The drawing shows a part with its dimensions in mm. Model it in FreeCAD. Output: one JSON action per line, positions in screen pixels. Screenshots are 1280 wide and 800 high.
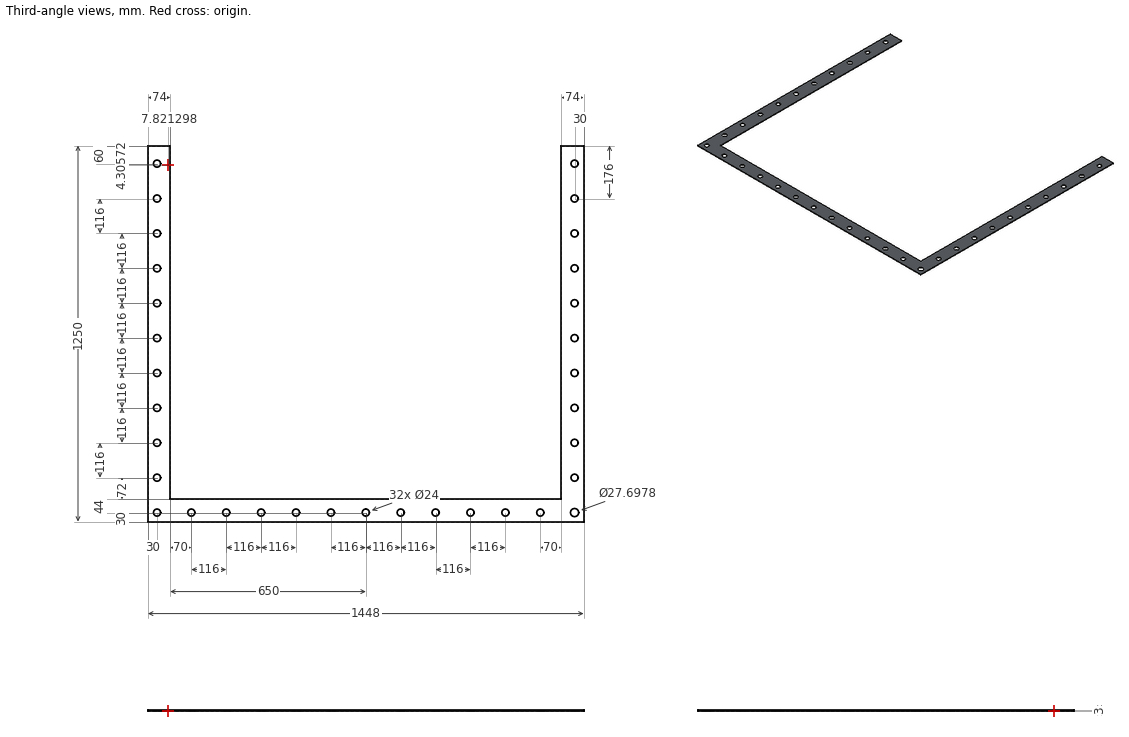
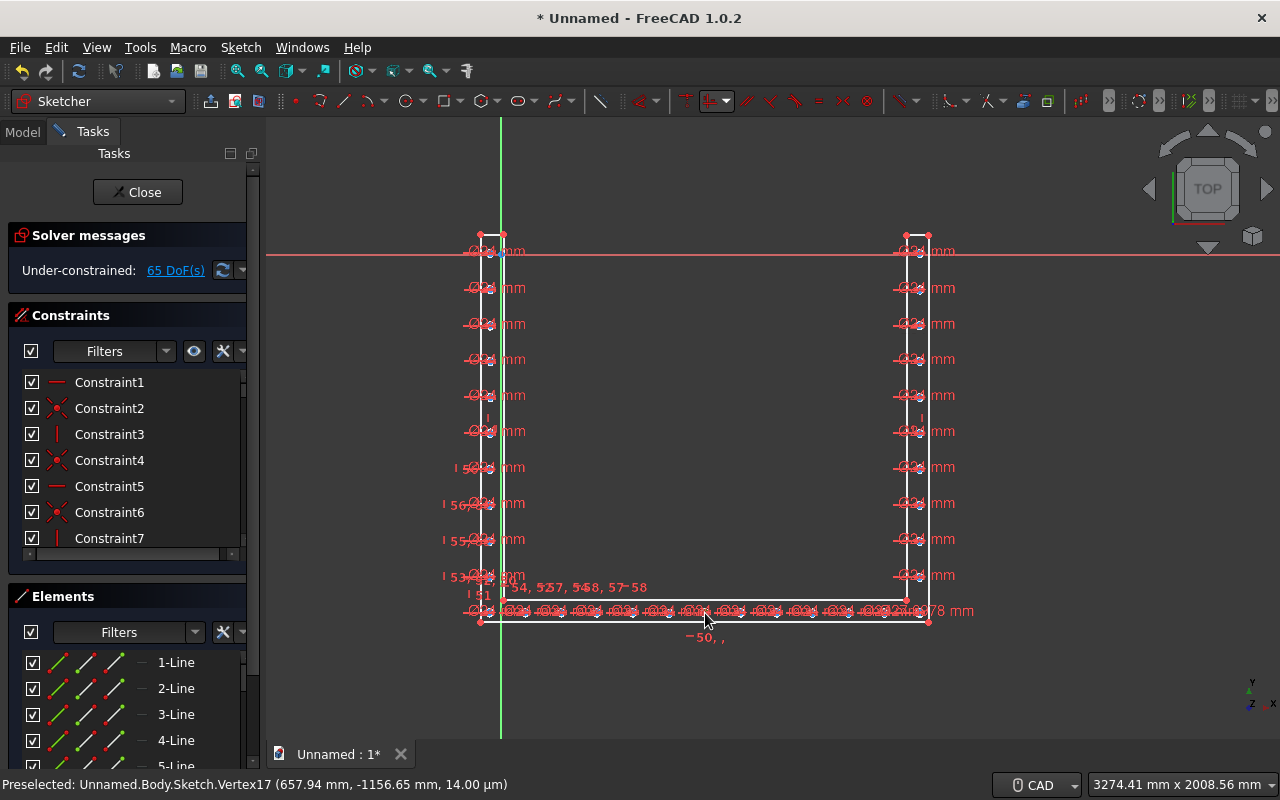
{"action": "left_click", "coordinate": [669, 613]}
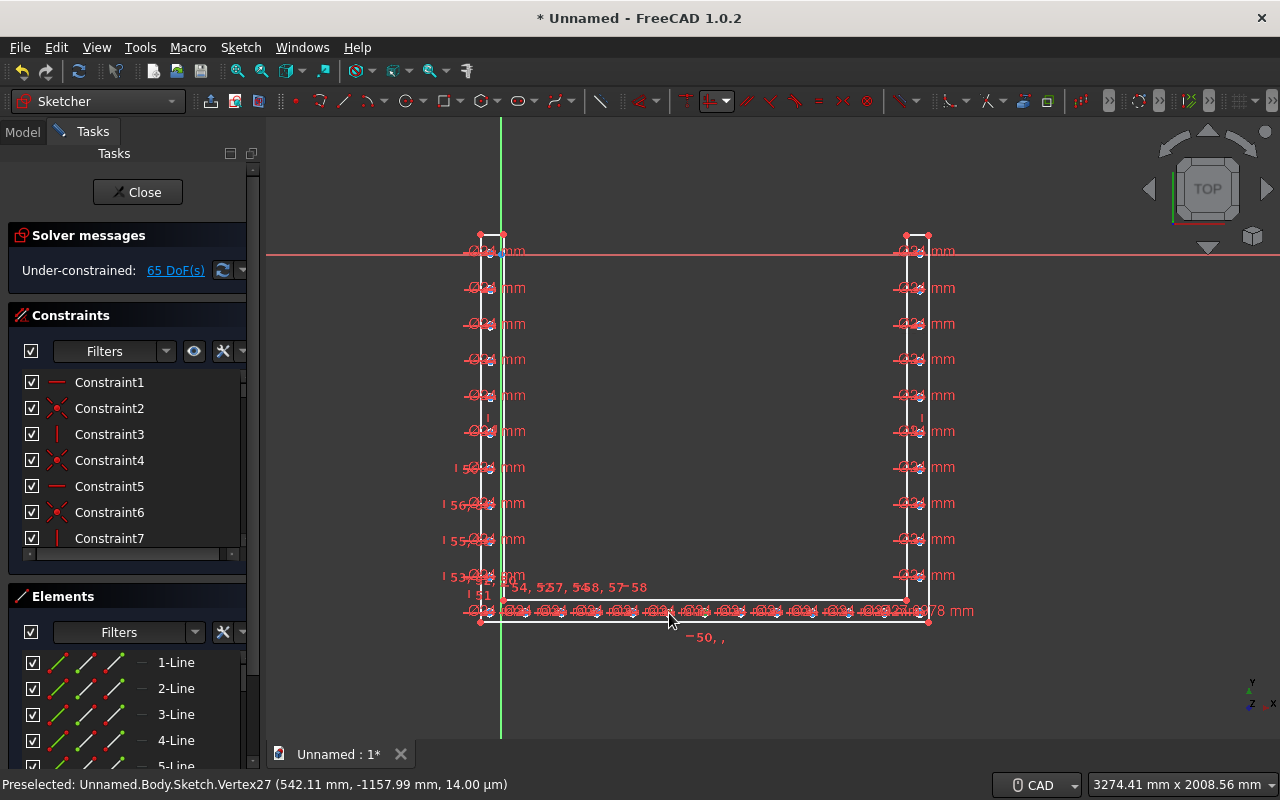
{"action": "left_click", "coordinate": [728, 102]}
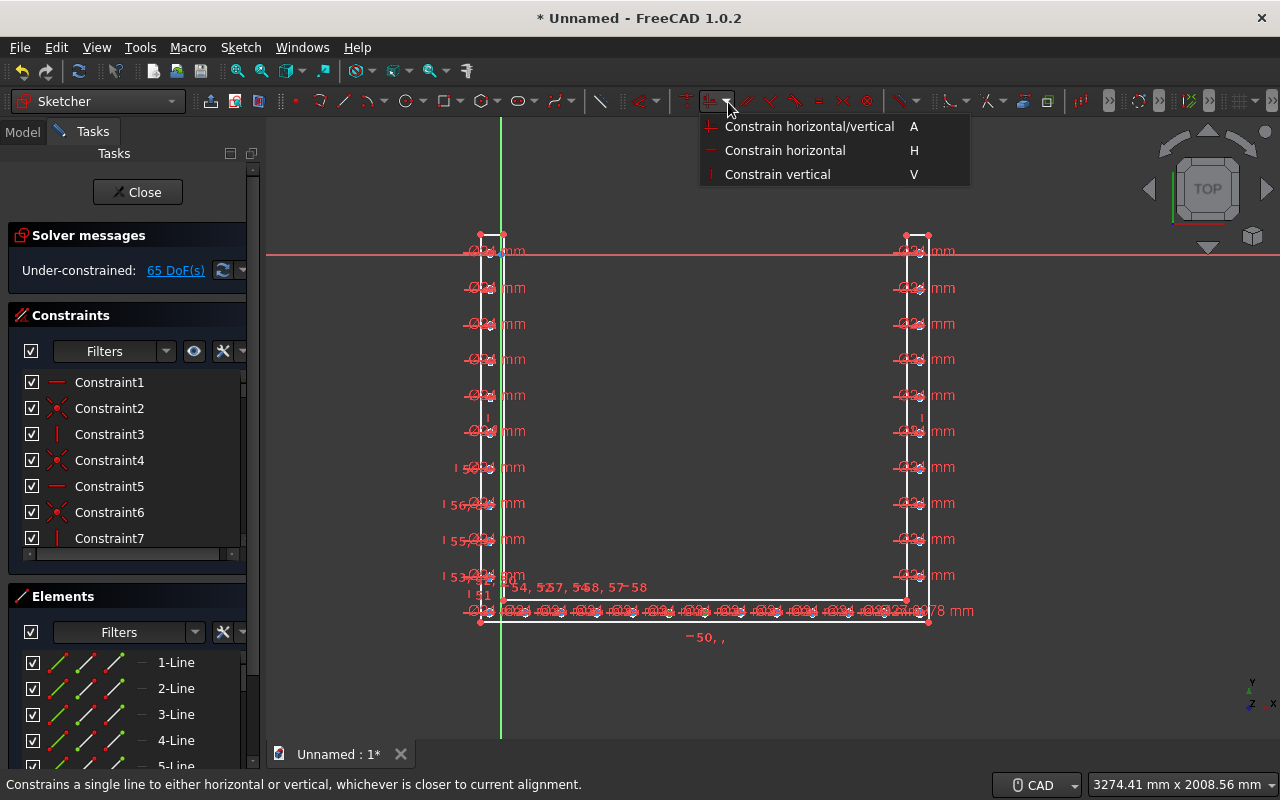
{"action": "left_click", "coordinate": [835, 150]}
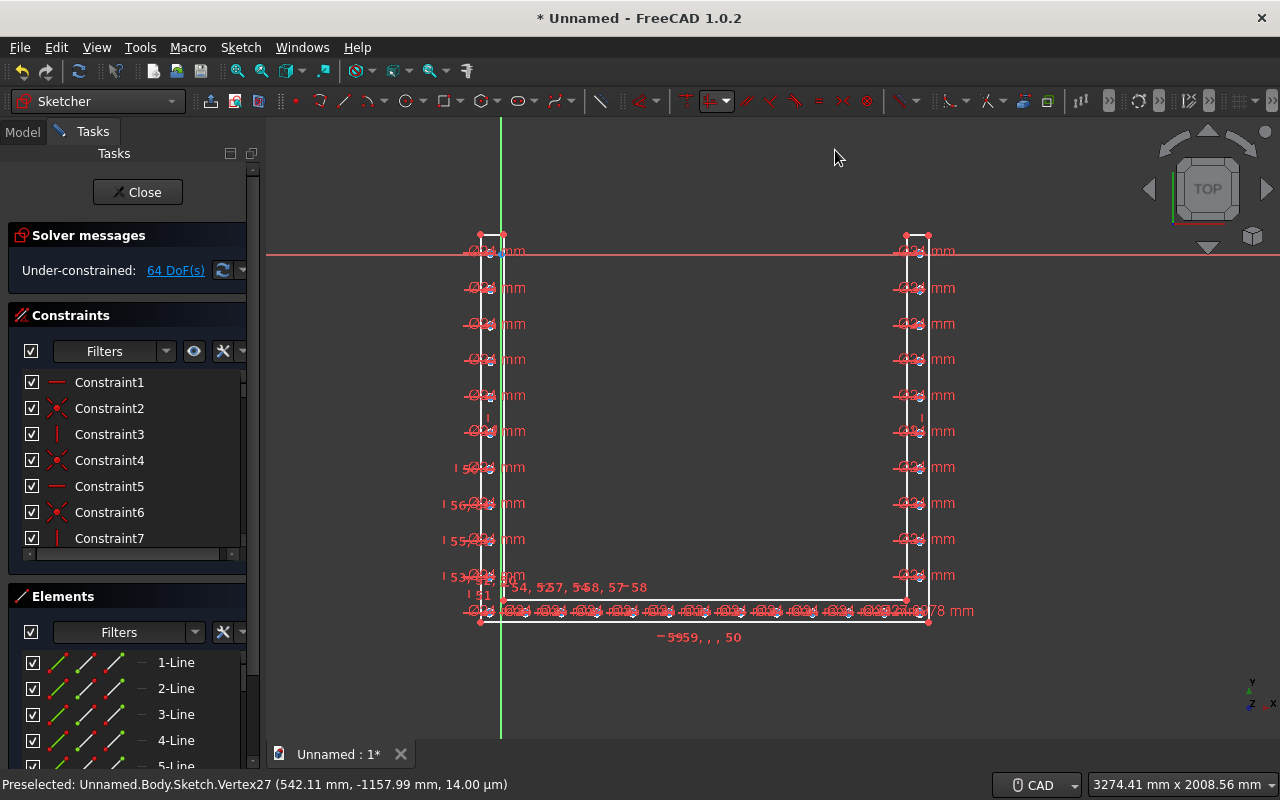
{"action": "left_click", "coordinate": [490, 469]}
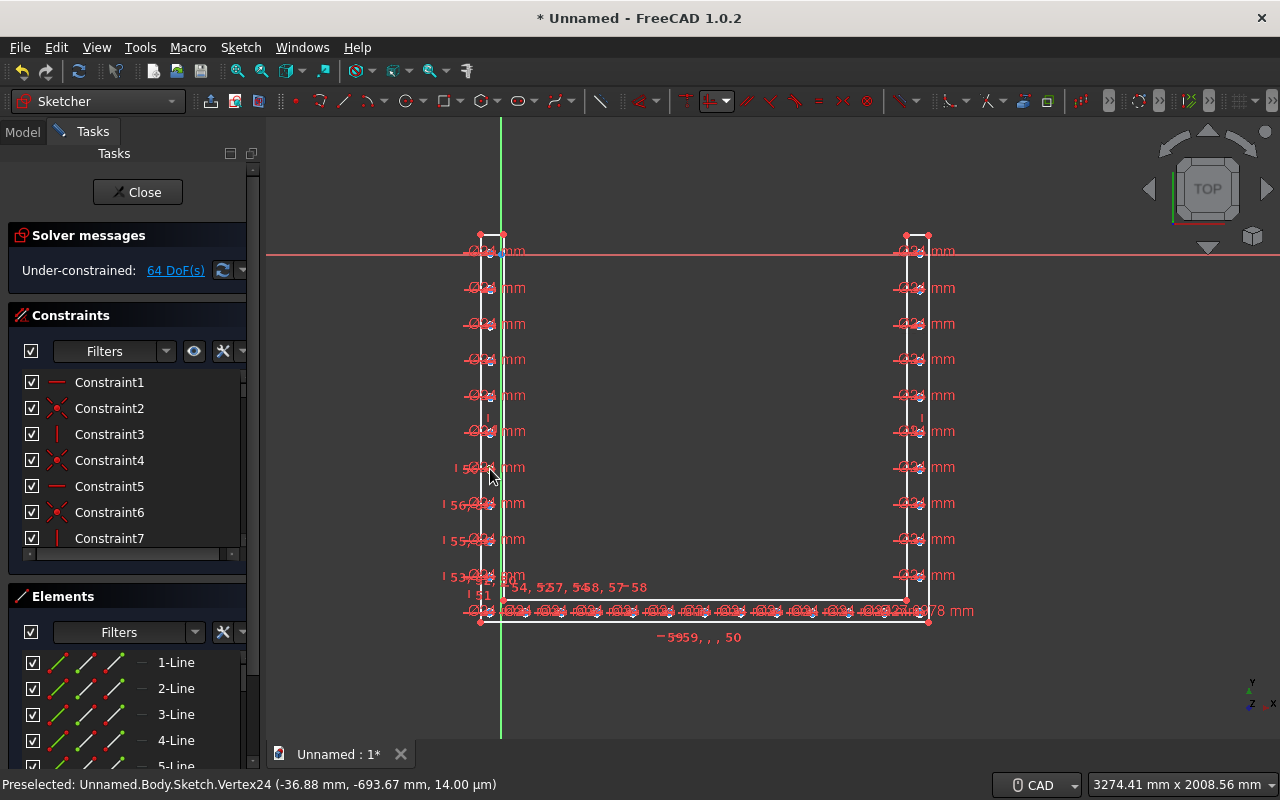
{"action": "left_click", "coordinate": [490, 433]}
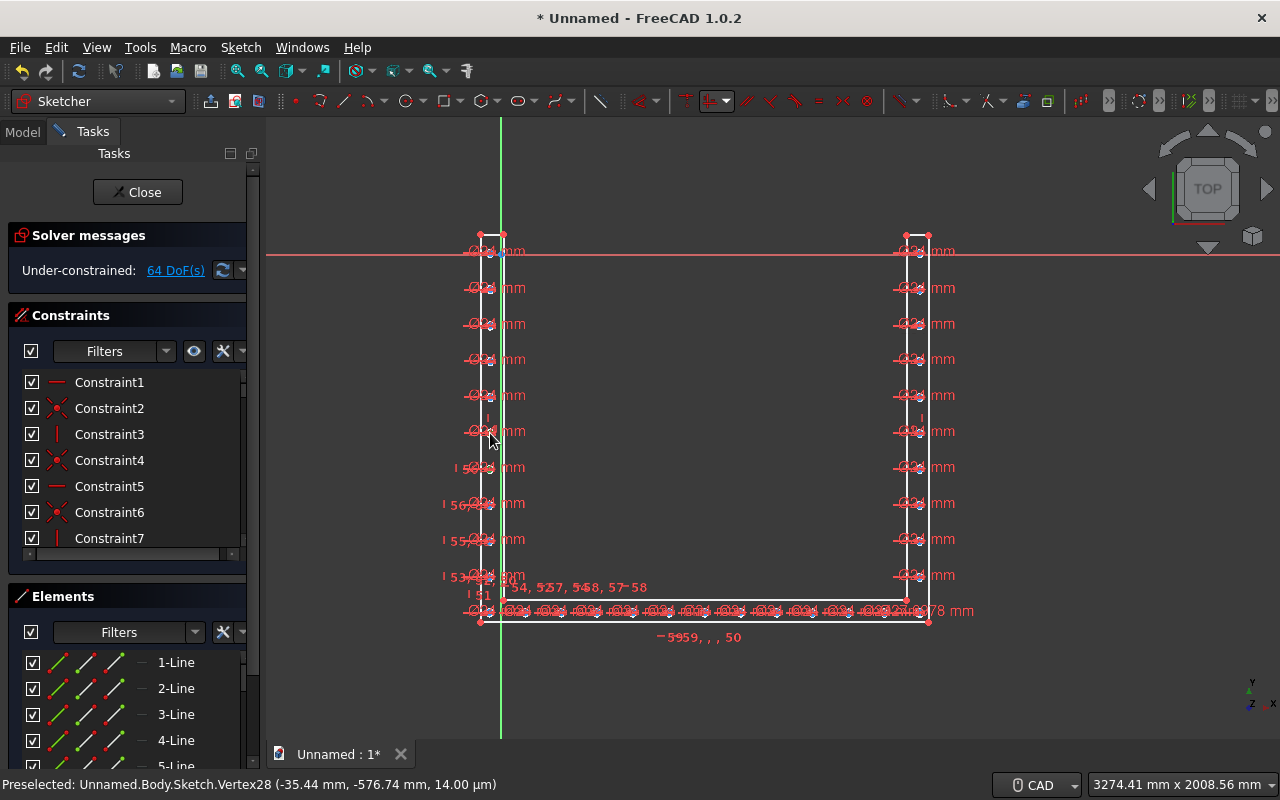
{"action": "key", "text": "v"}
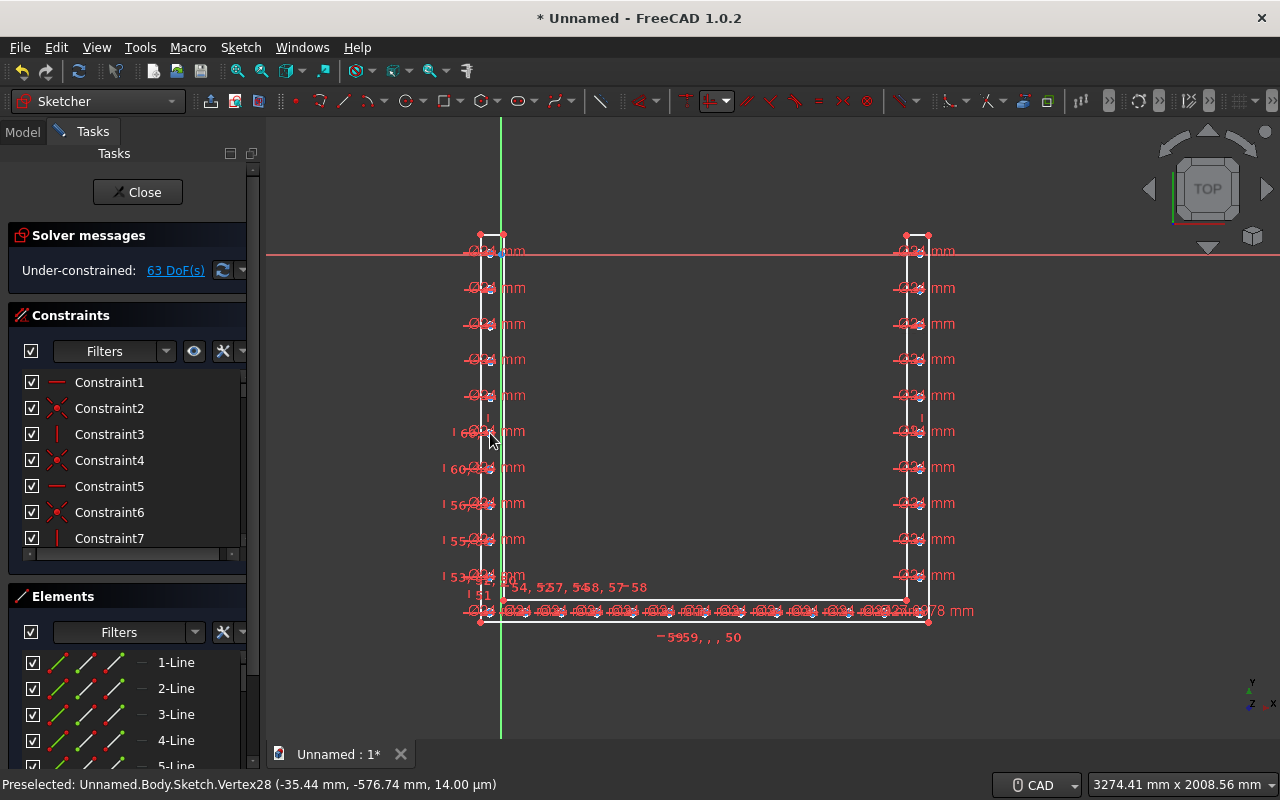
{"action": "left_click", "coordinate": [490, 433]}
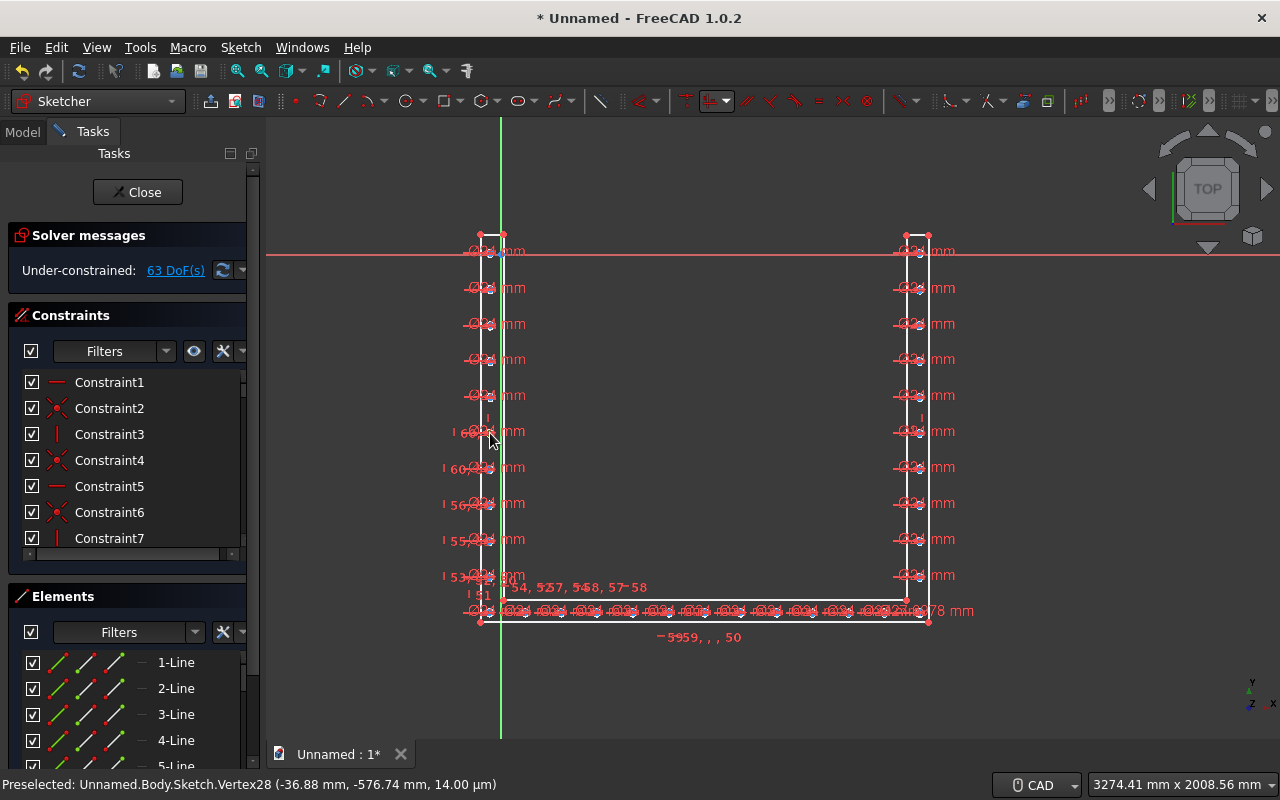
{"action": "left_click", "coordinate": [490, 397]}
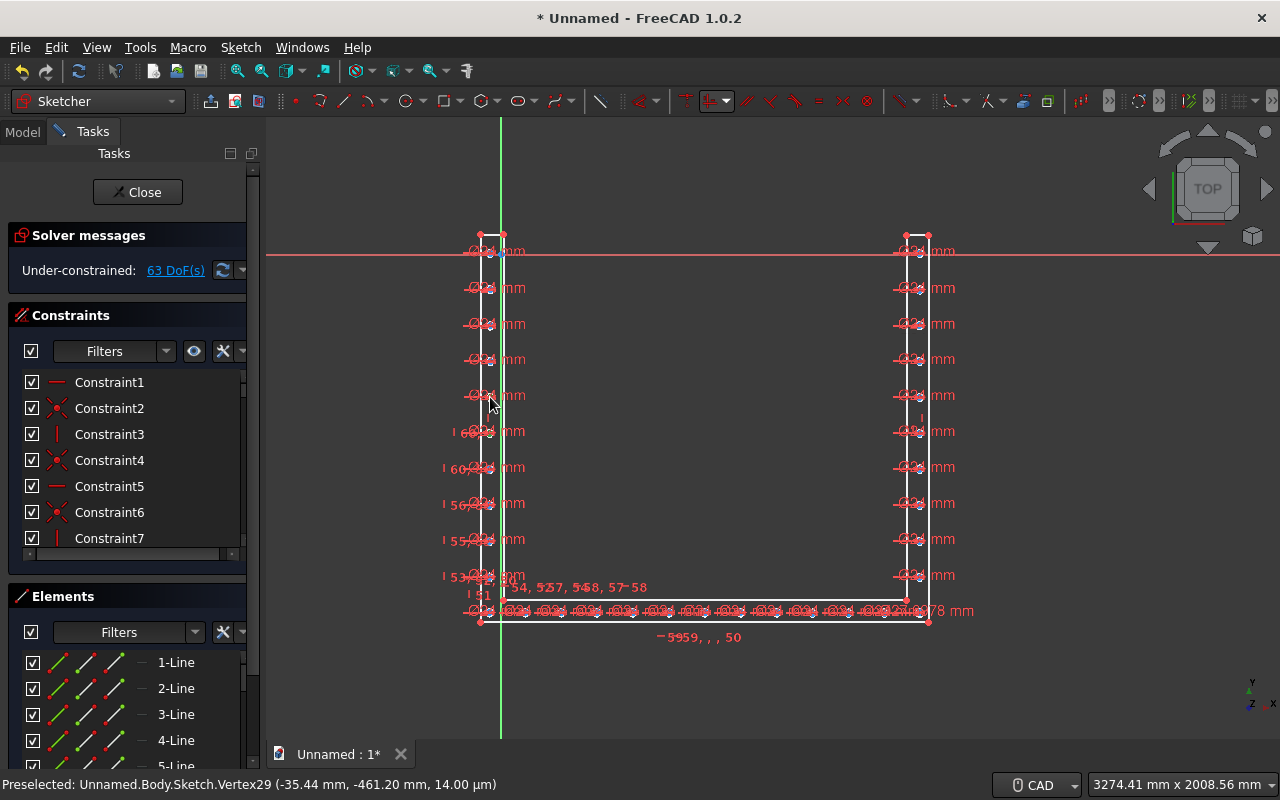
{"action": "left_click", "coordinate": [728, 102]}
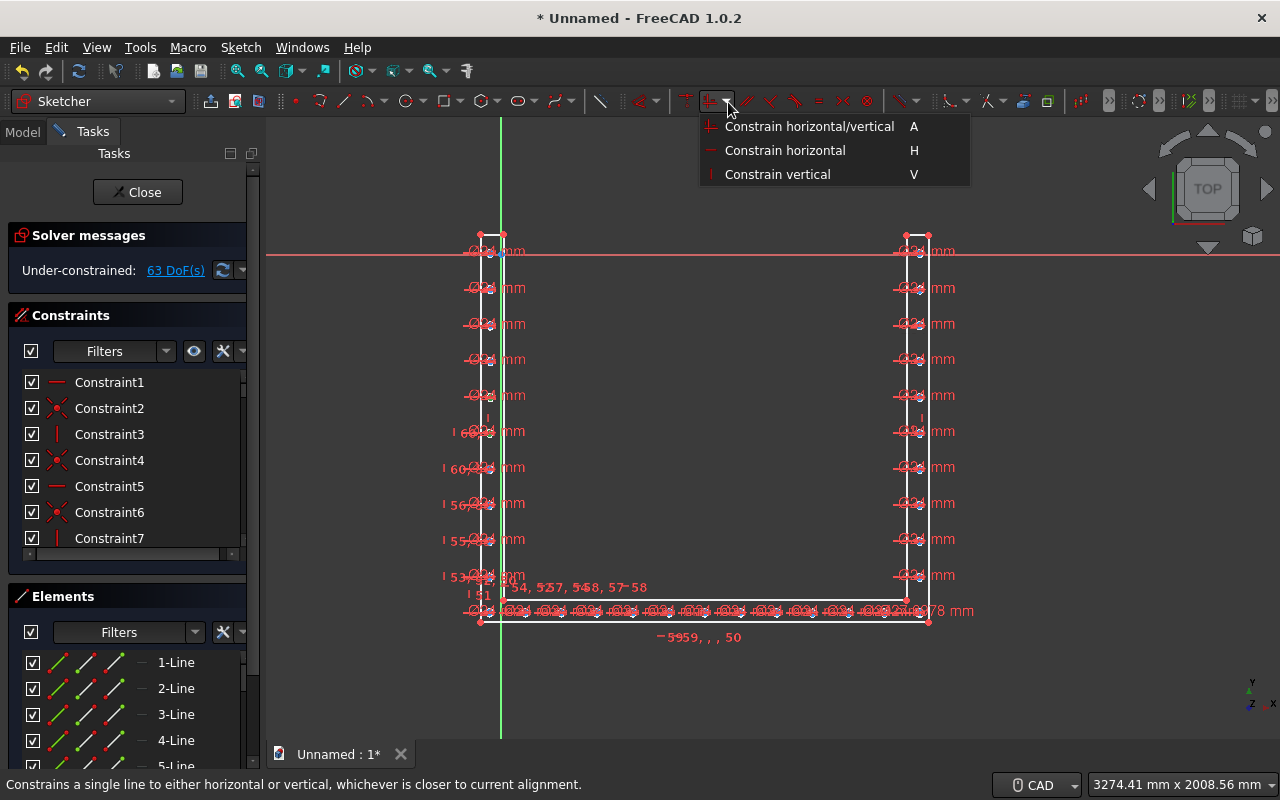
{"action": "left_click", "coordinate": [835, 174]}